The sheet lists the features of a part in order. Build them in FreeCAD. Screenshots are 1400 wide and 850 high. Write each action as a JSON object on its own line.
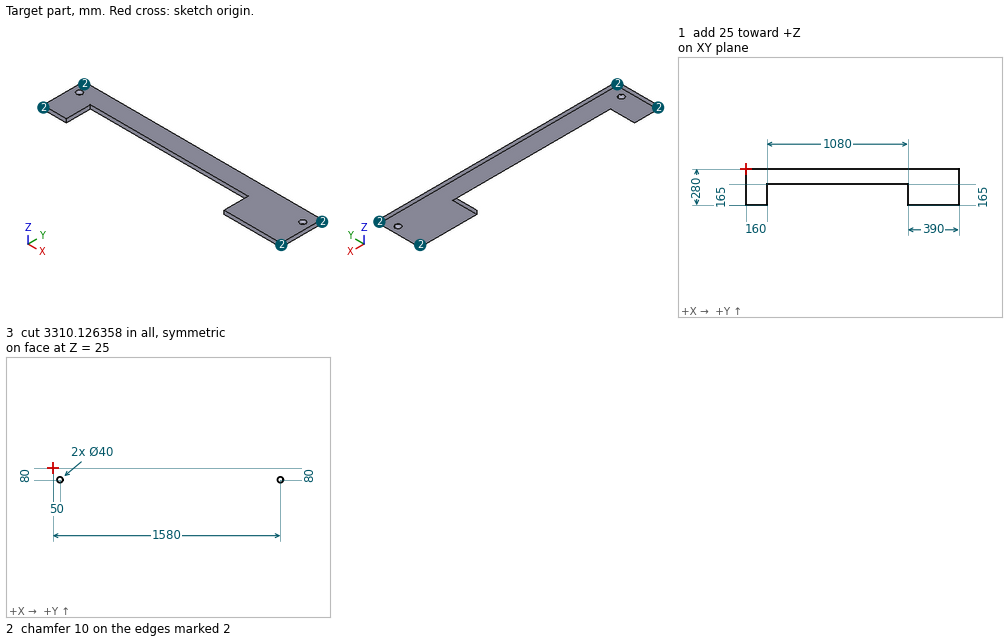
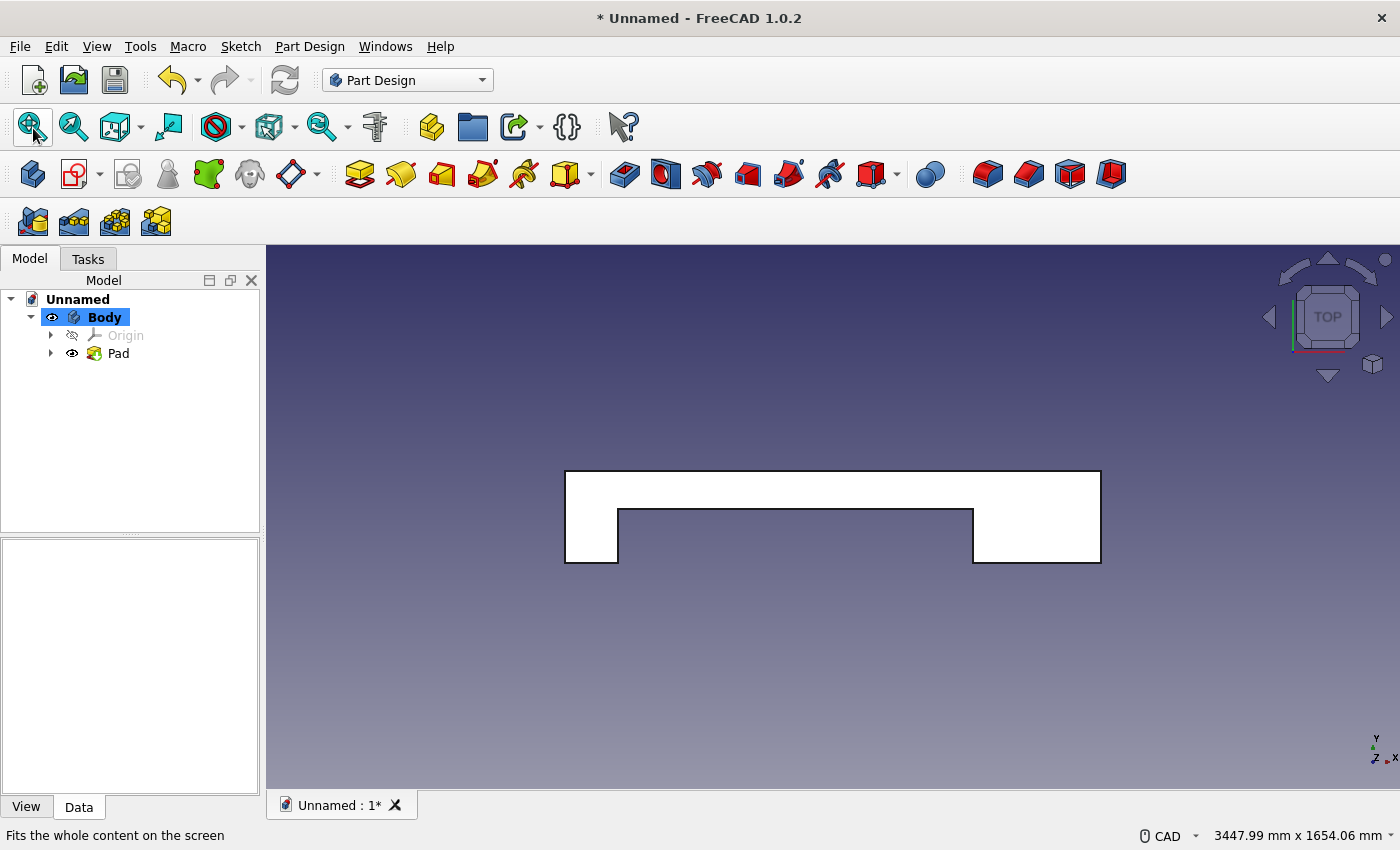
{"action": "key", "text": "1"}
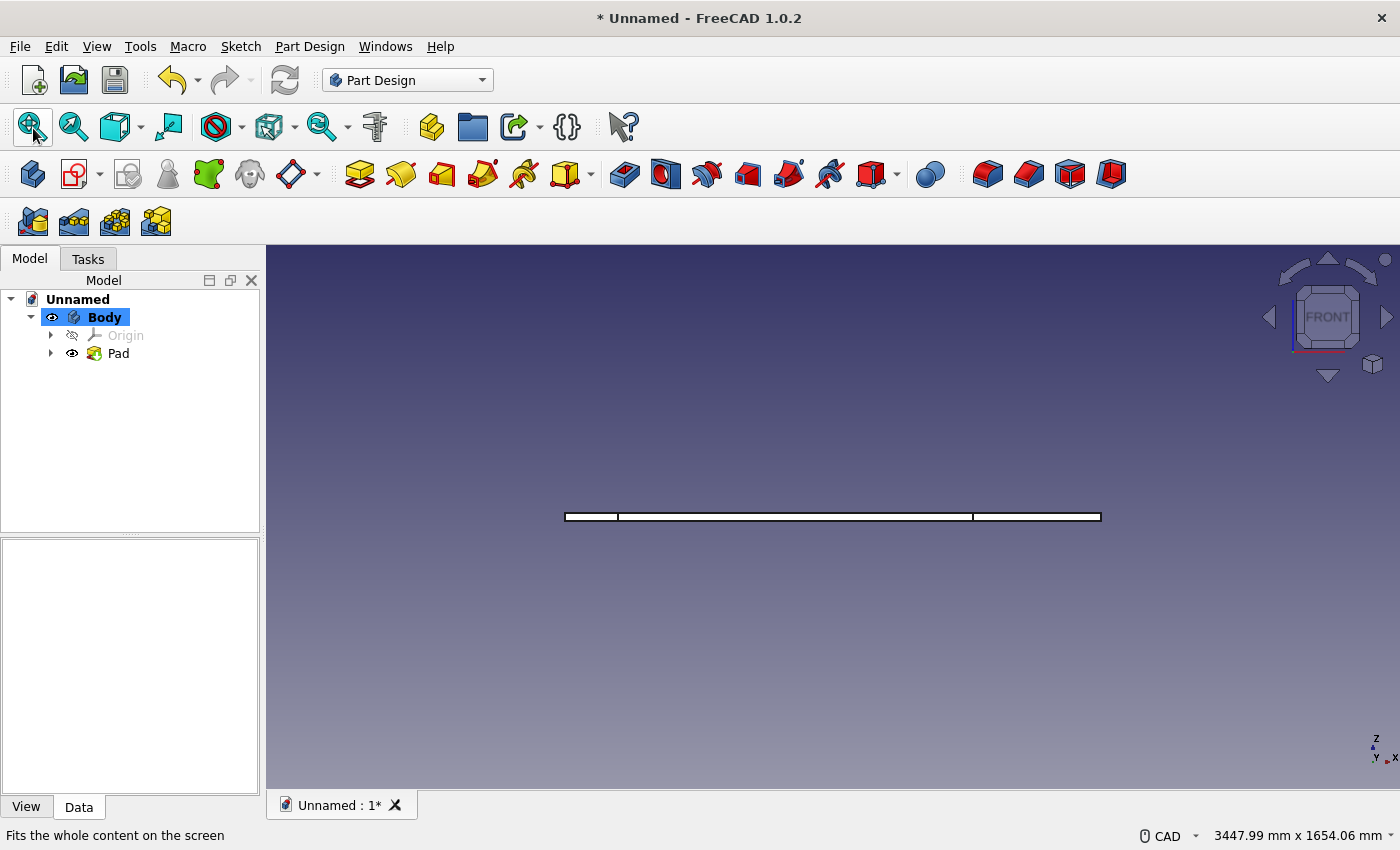
{"action": "scroll", "coordinate": [565, 516], "scroll_direction": "up", "scroll_amount": 8}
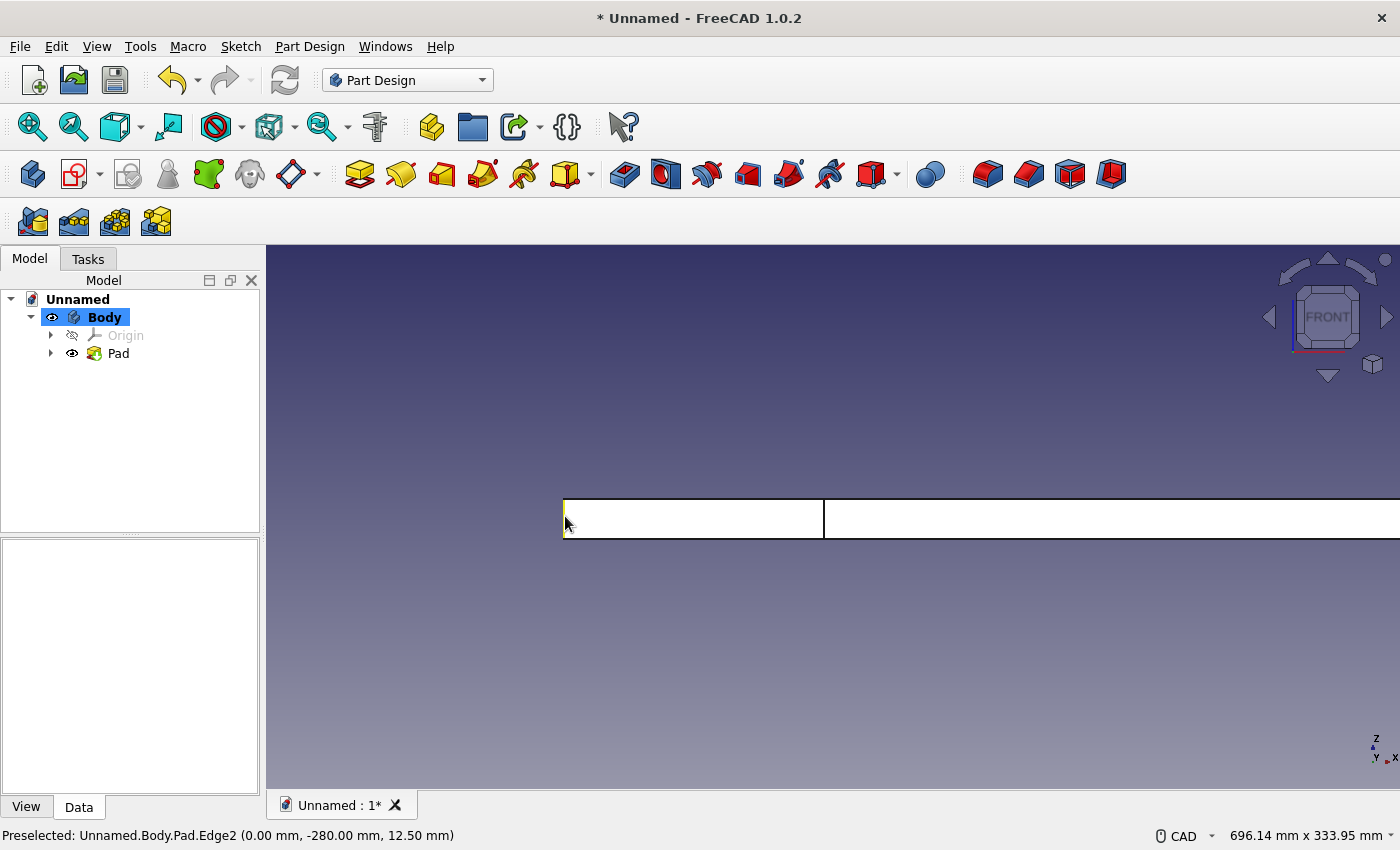
{"action": "left_click", "coordinate": [564, 518]}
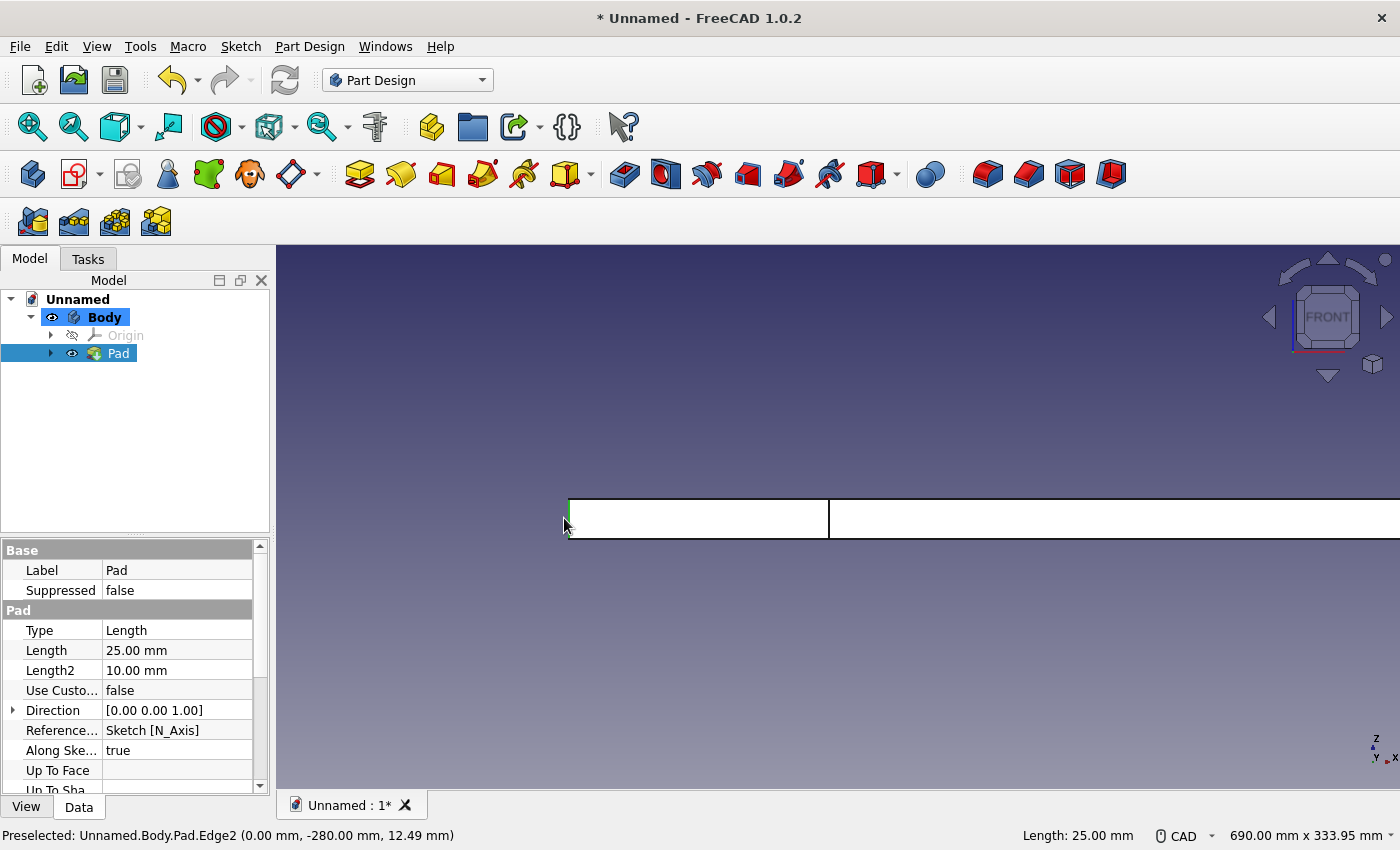
{"action": "key", "text": "v f"}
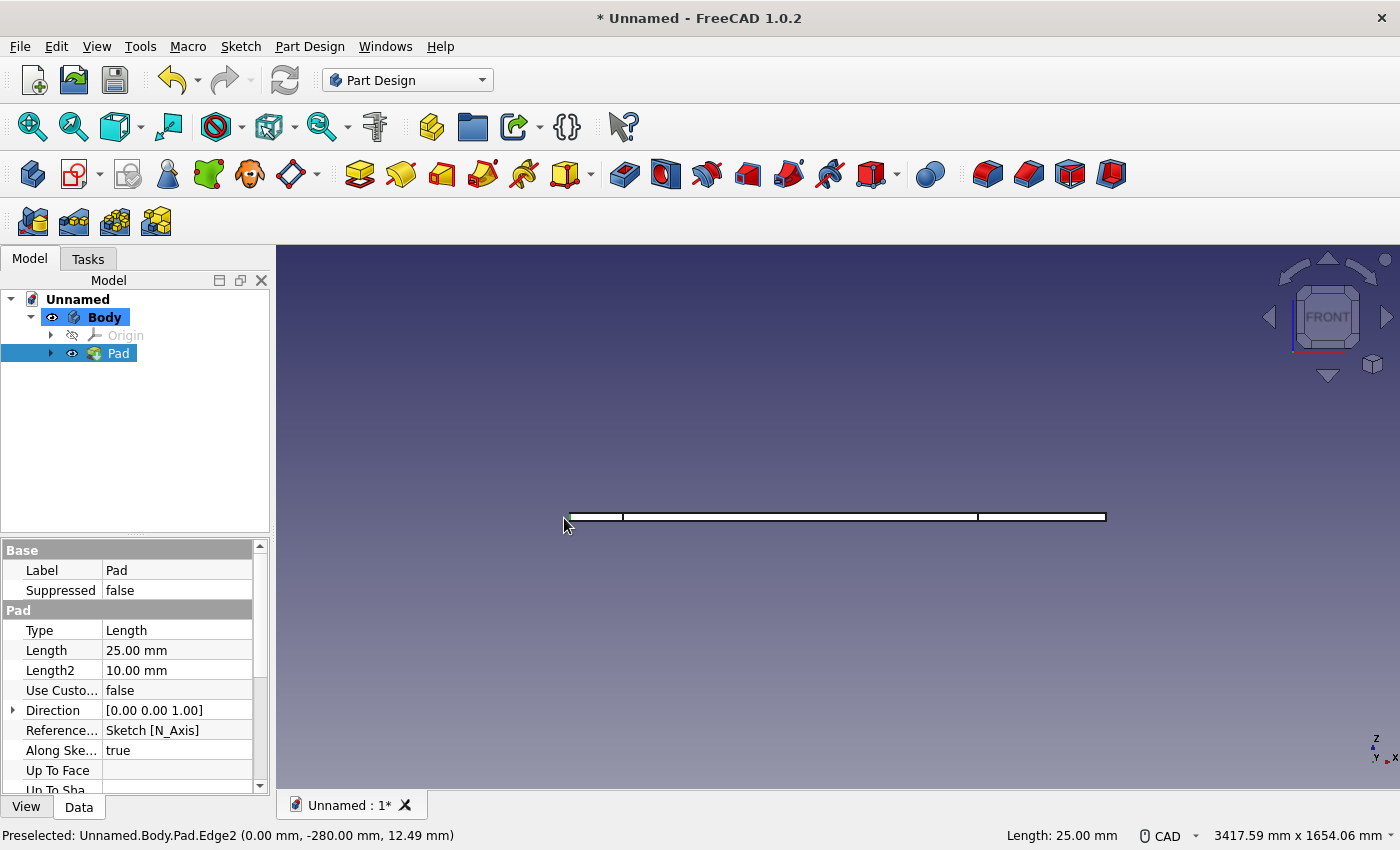
{"action": "key", "text": "3"}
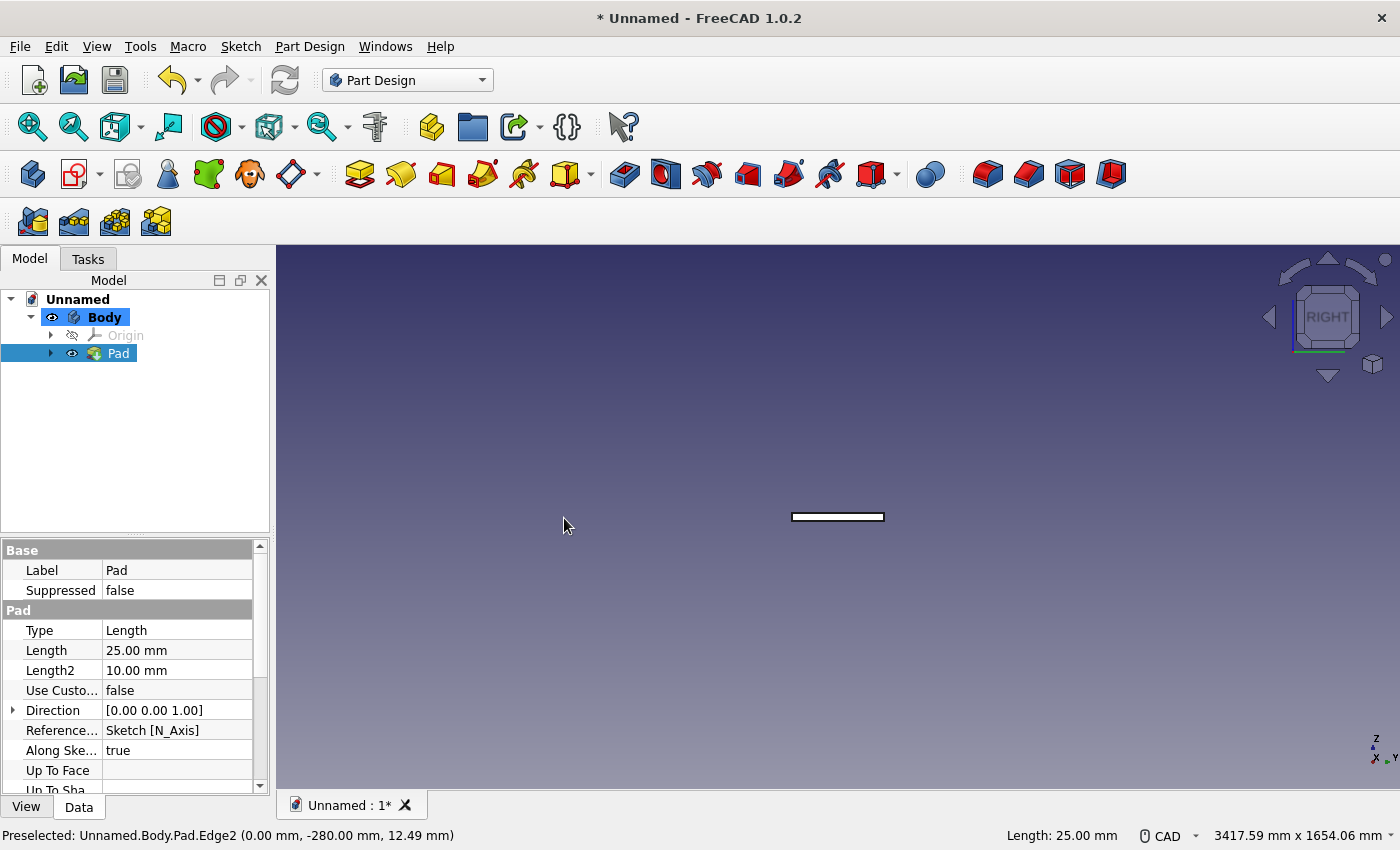
{"action": "key", "text": "v f"}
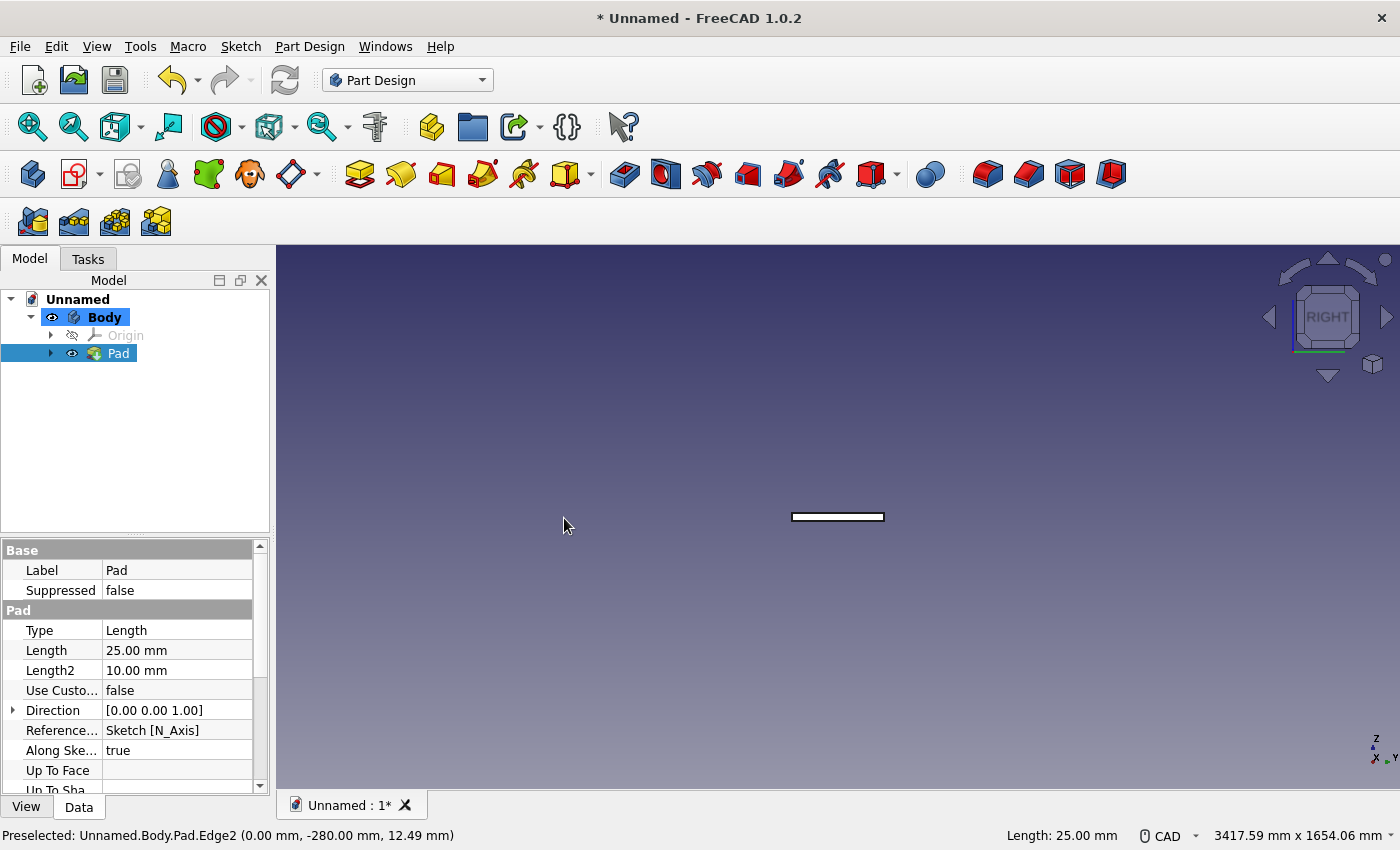
{"action": "scroll", "coordinate": [884, 516], "scroll_direction": "up", "scroll_amount": 8}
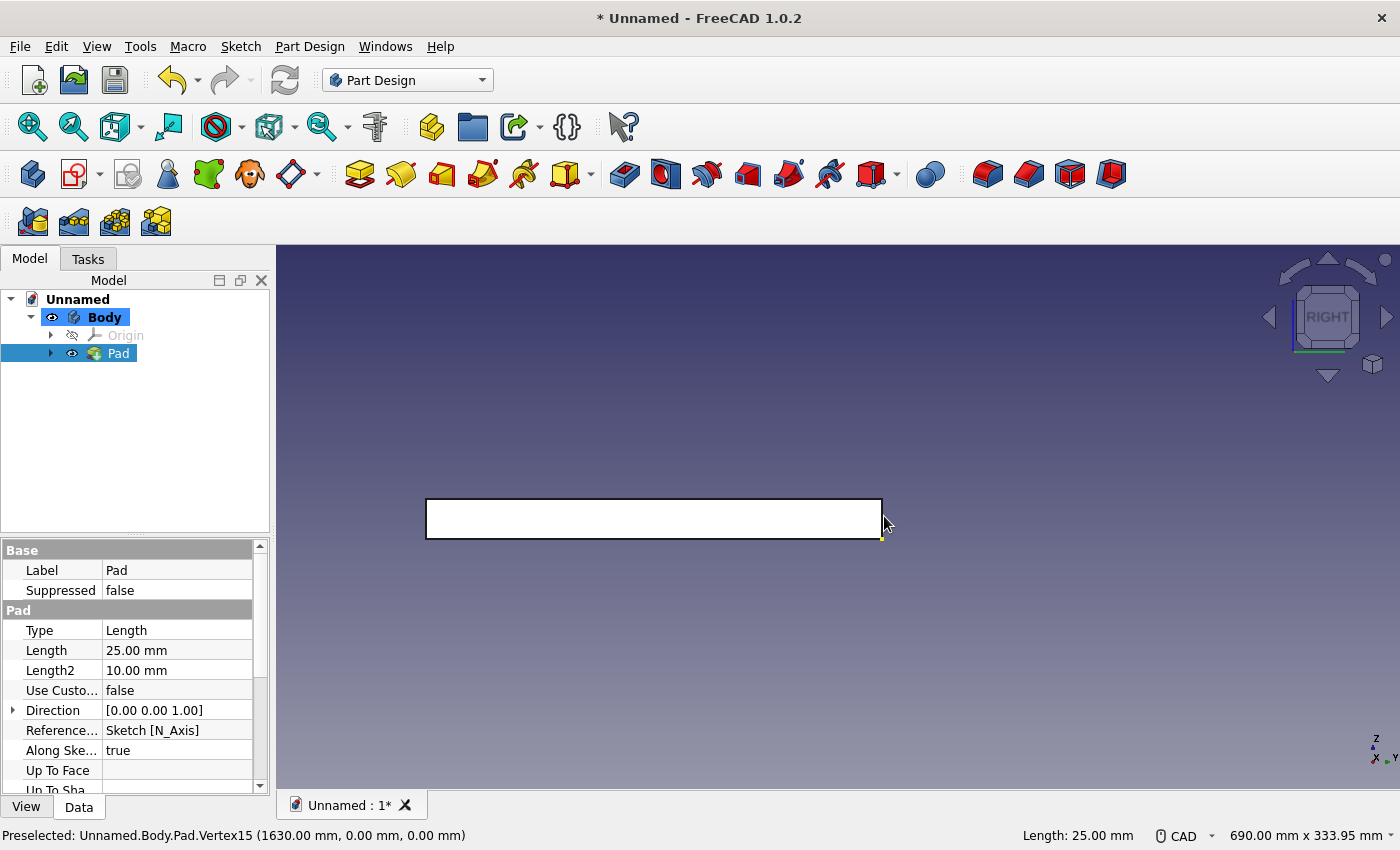
{"action": "left_click", "coordinate": [882, 518], "text": "ctrl"}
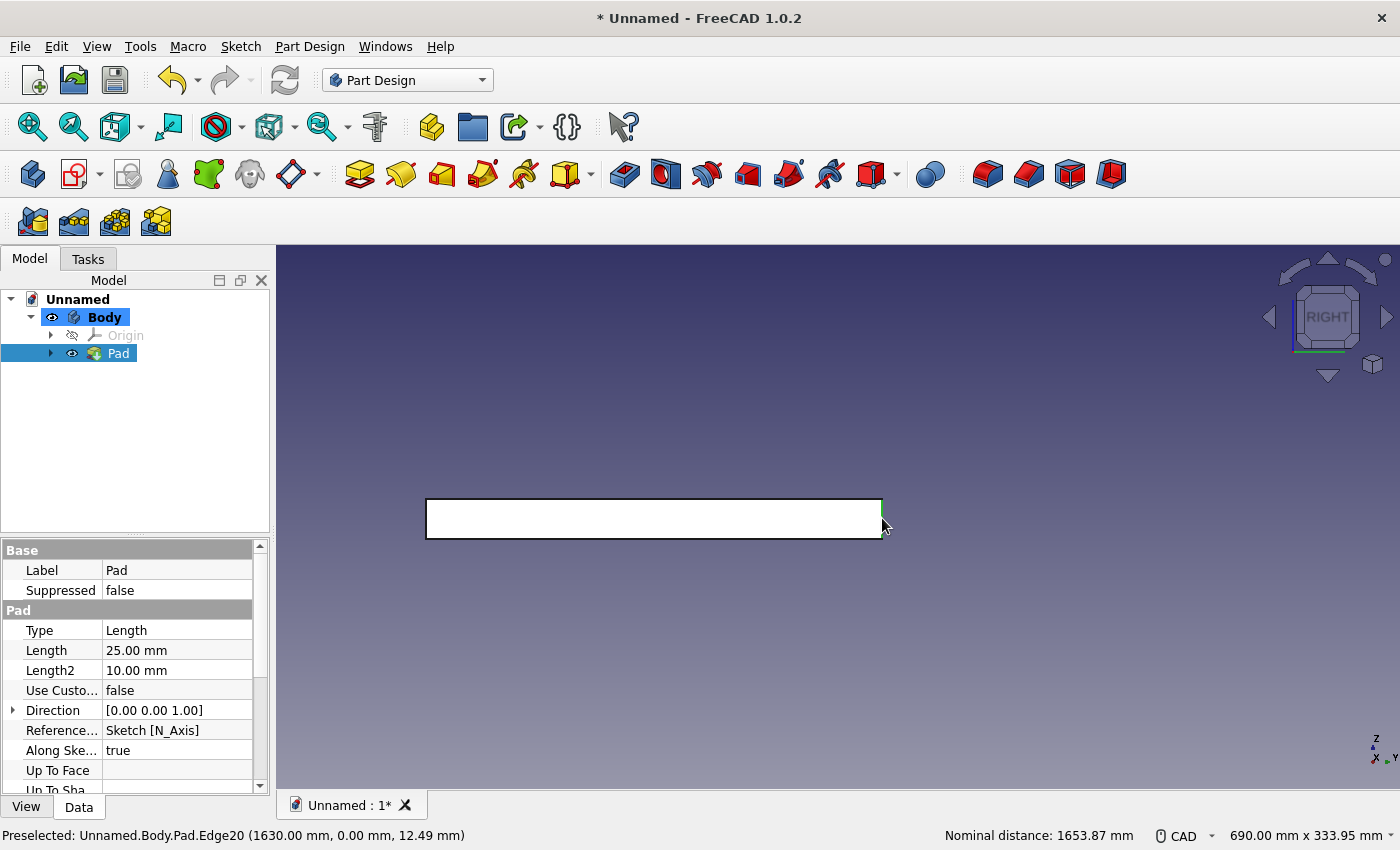
{"action": "left_click", "coordinate": [426, 518], "text": "ctrl"}